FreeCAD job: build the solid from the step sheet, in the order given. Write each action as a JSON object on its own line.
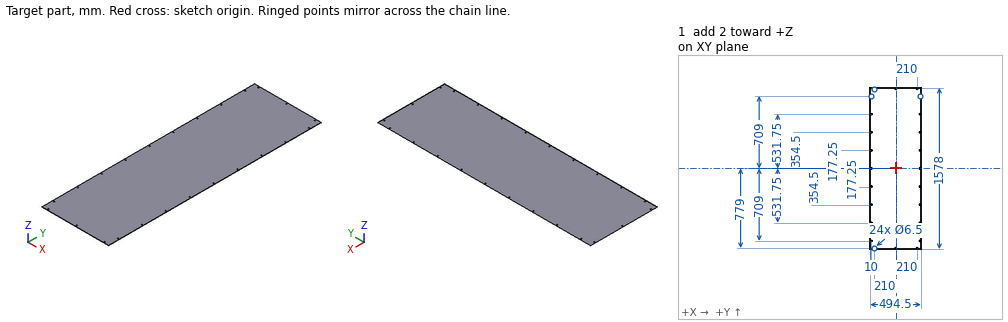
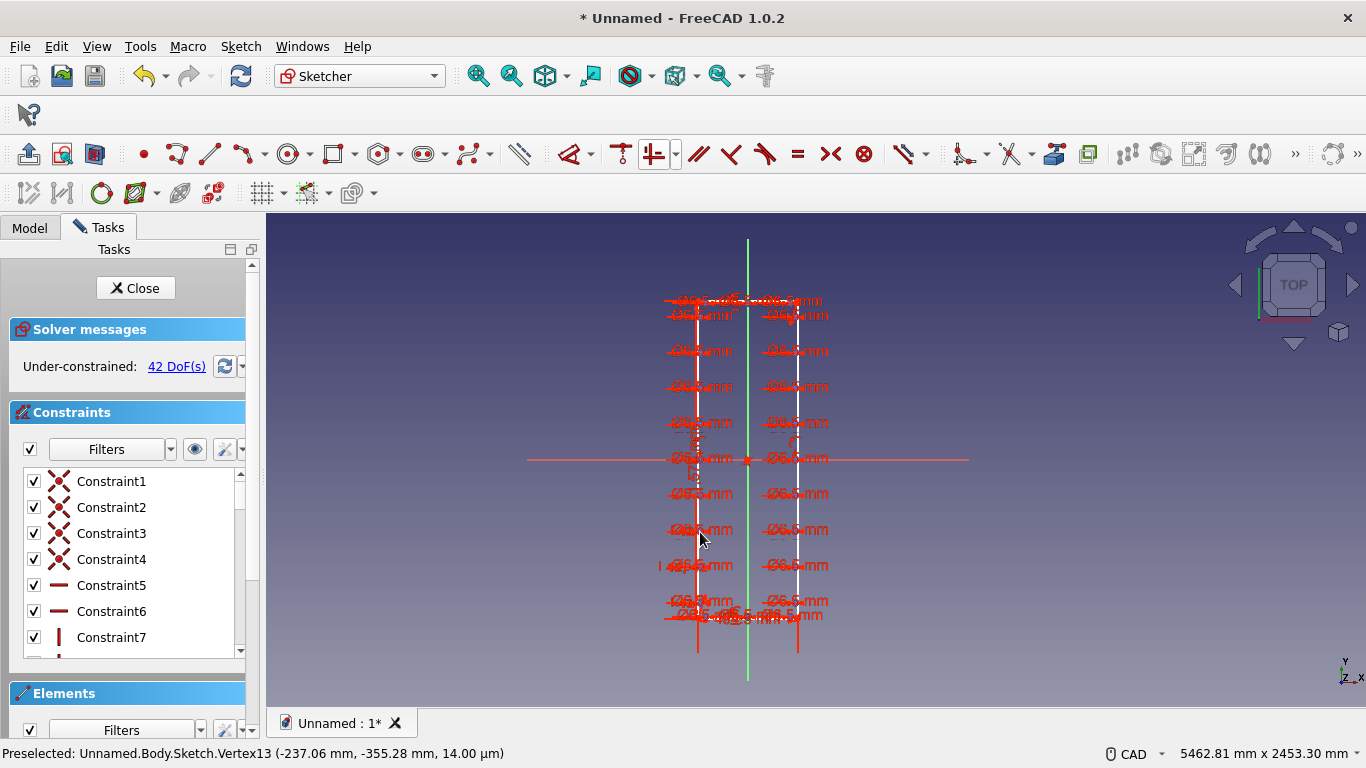
{"action": "left_click", "coordinate": [700, 532]}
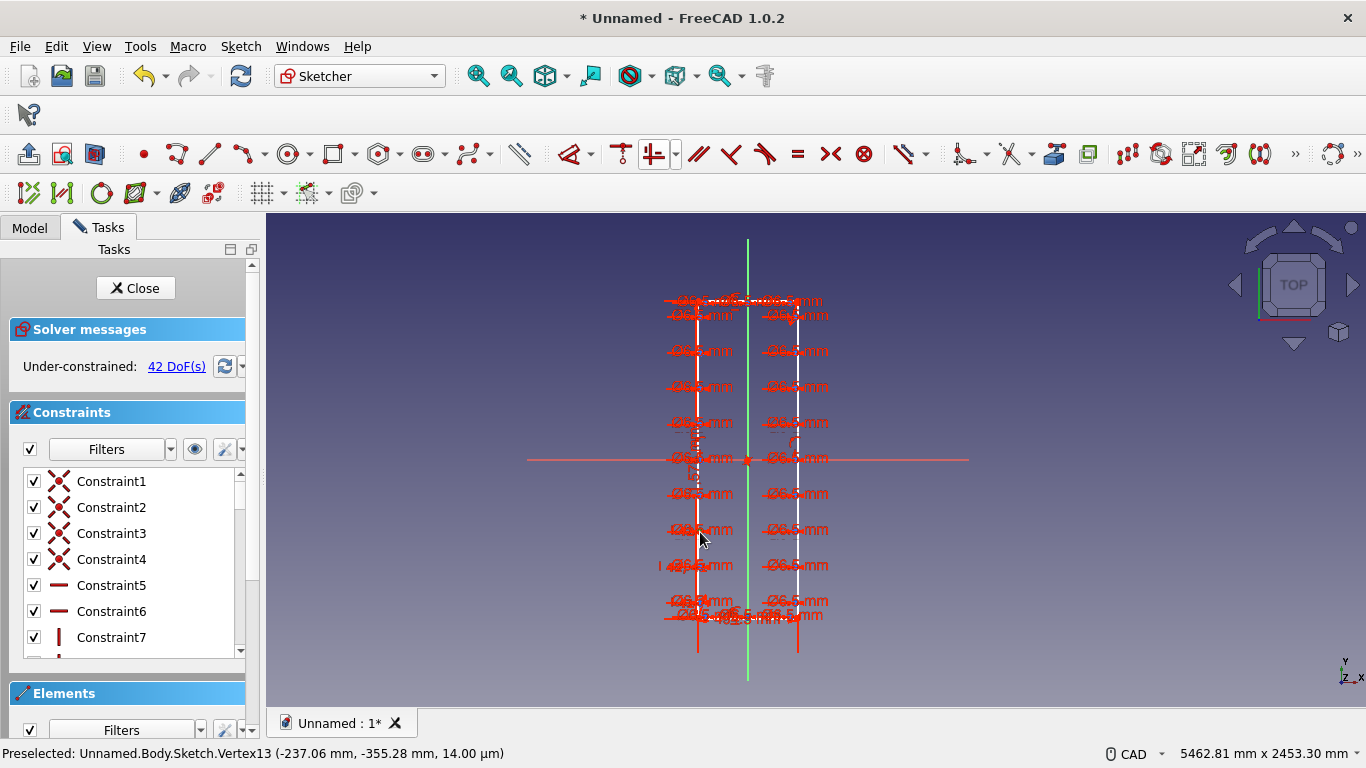
{"action": "left_click", "coordinate": [700, 496]}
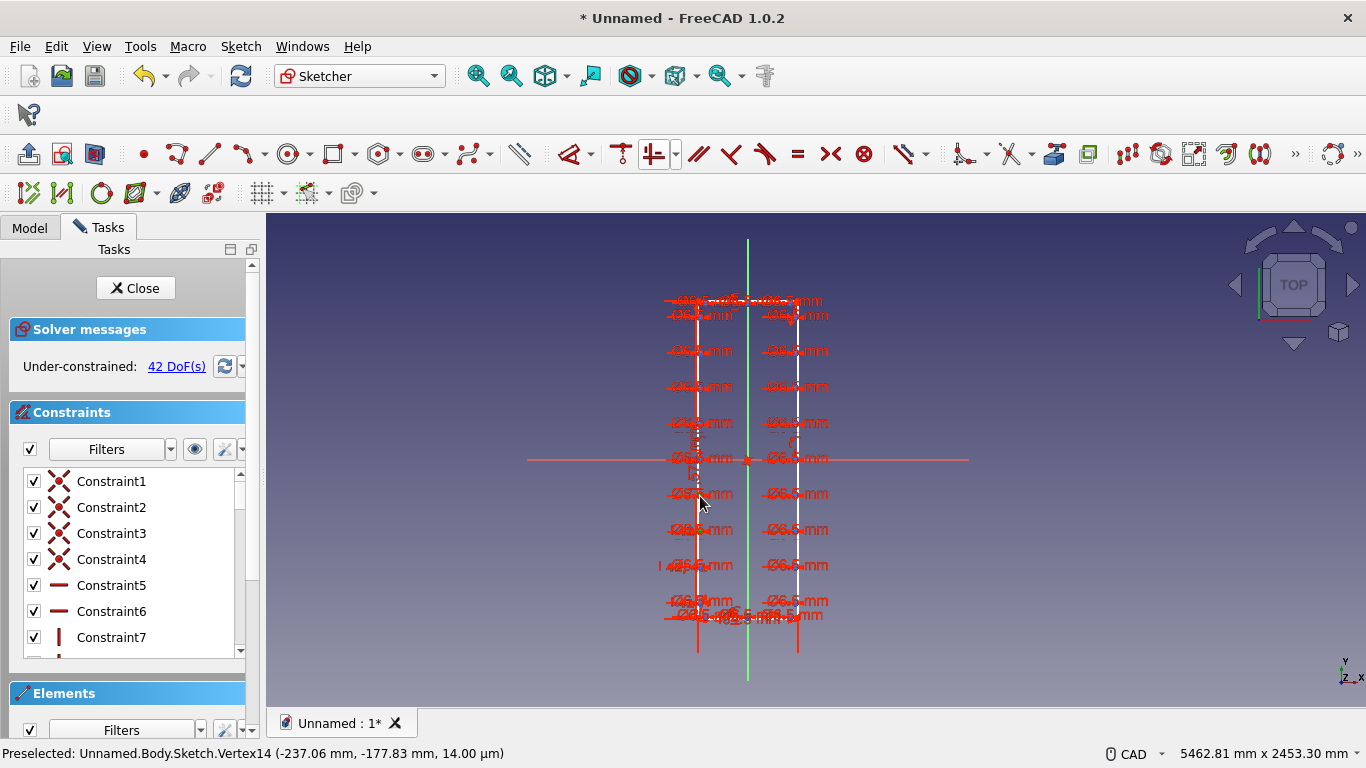
{"action": "left_click", "coordinate": [676, 154]}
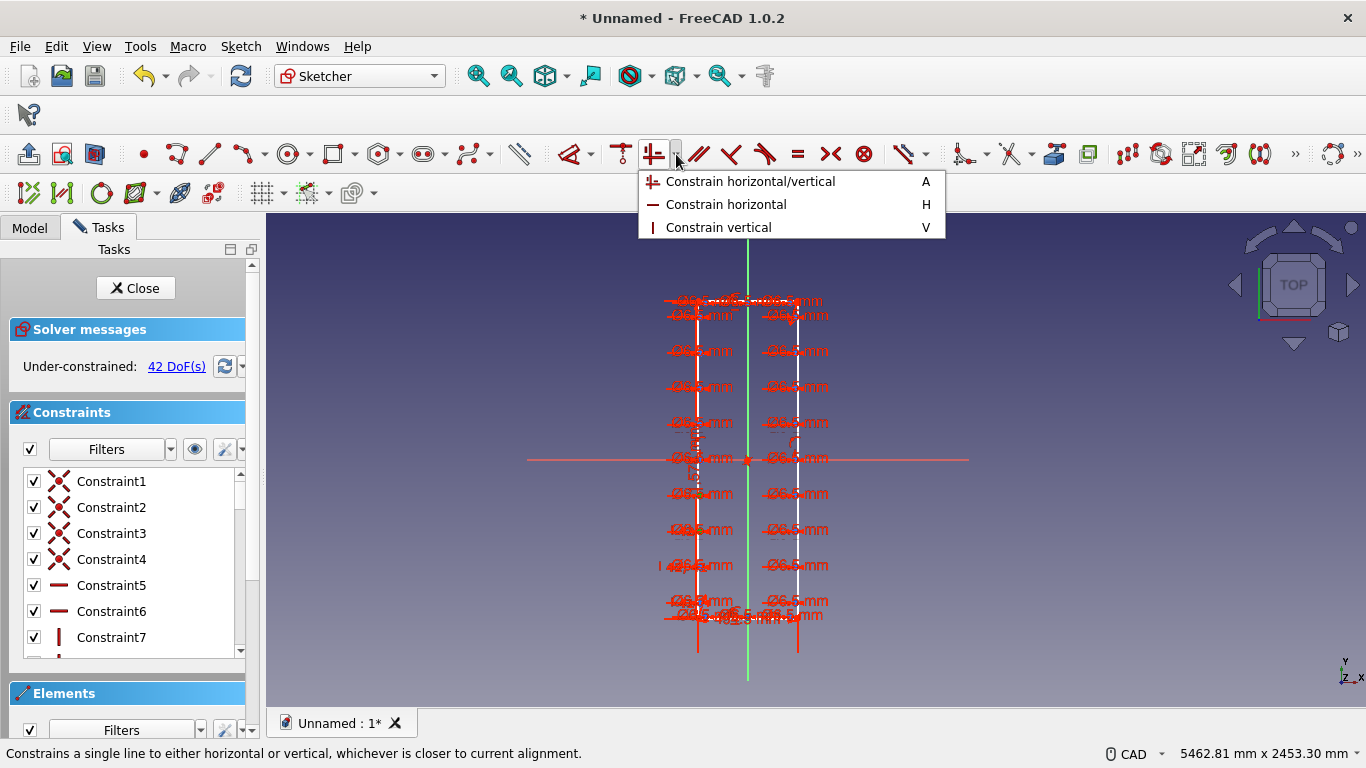
{"action": "left_click", "coordinate": [792, 228]}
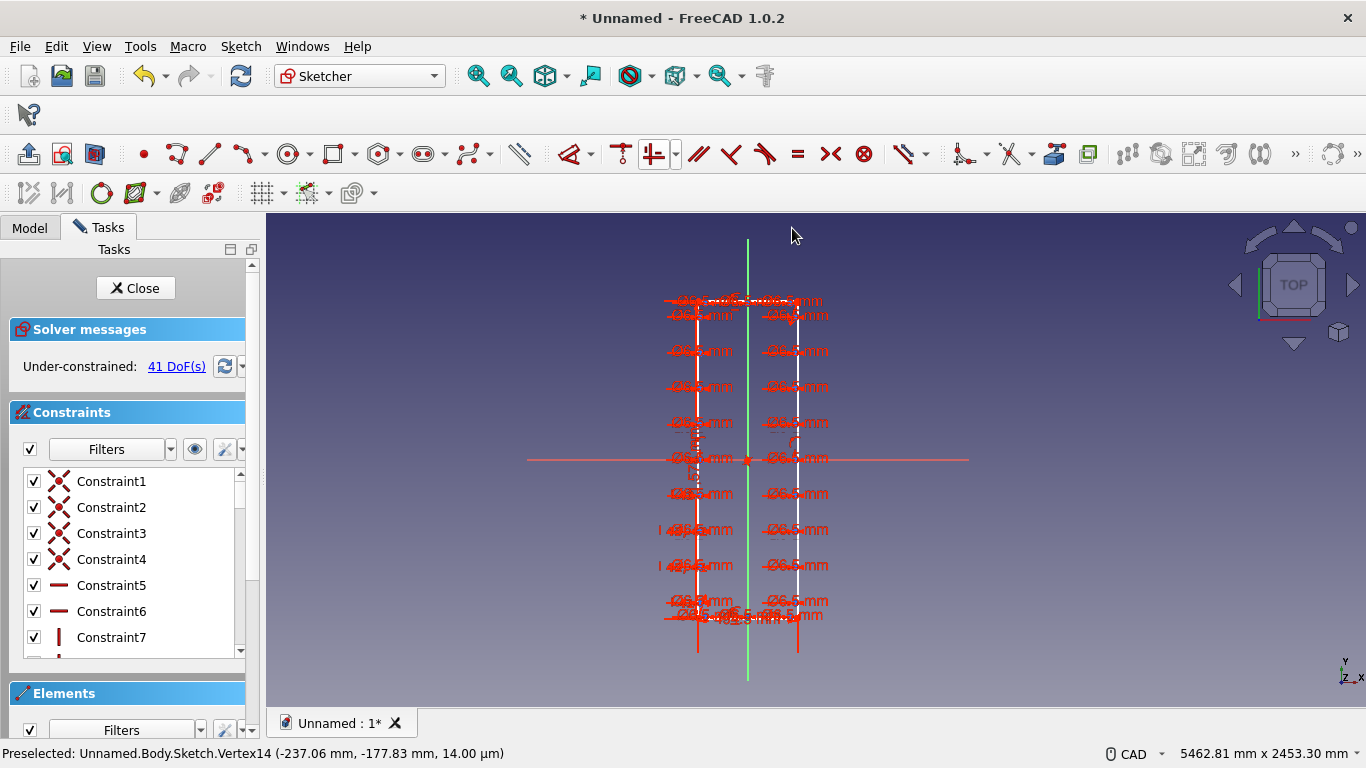
{"action": "scroll", "coordinate": [706, 617], "scroll_direction": "up", "scroll_amount": 3}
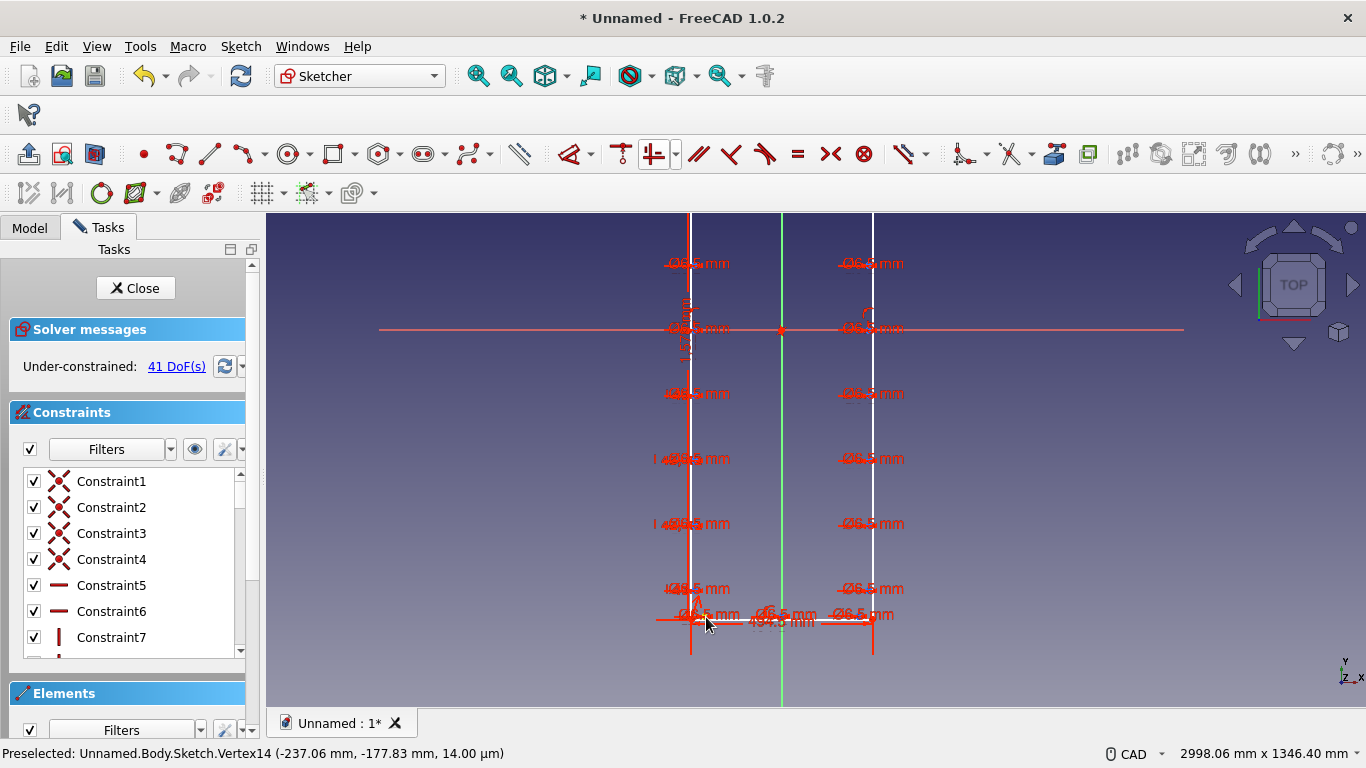
{"action": "left_click", "coordinate": [705, 617]}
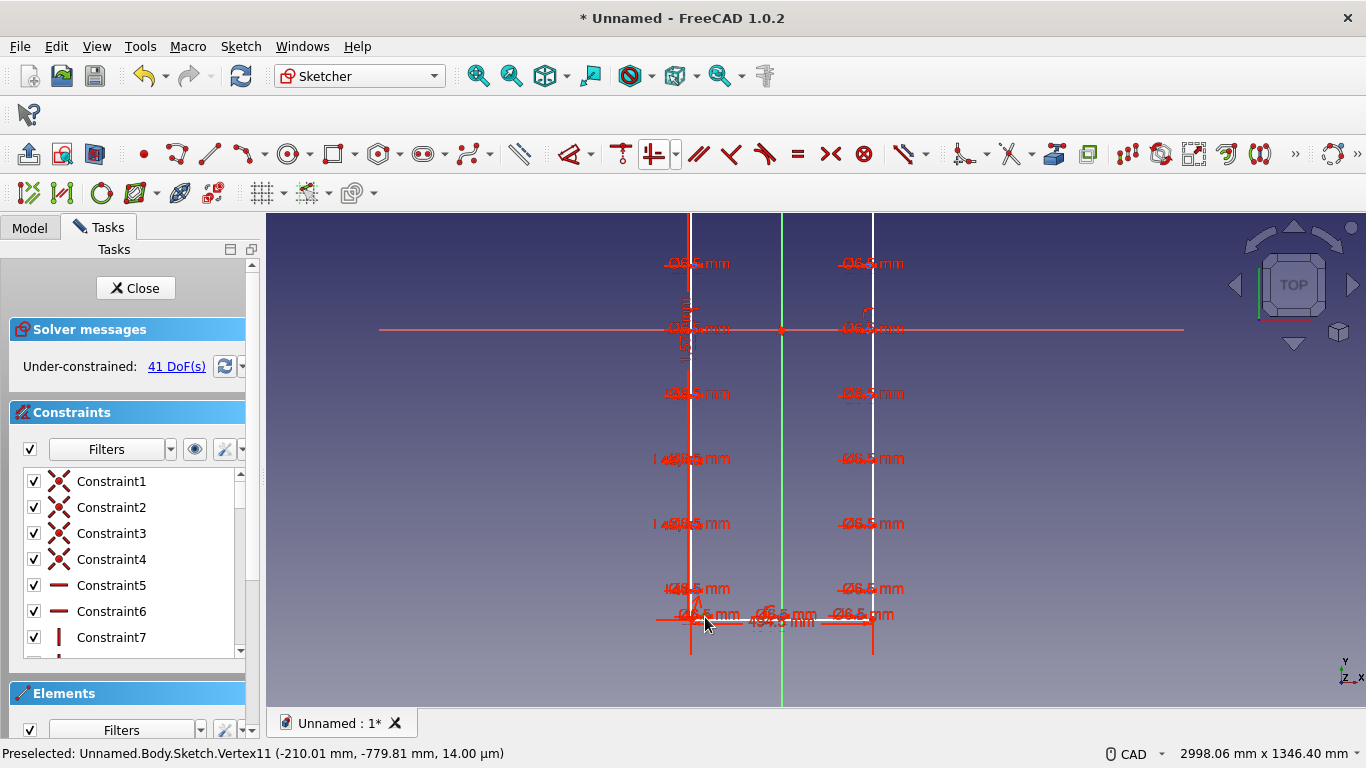
{"action": "left_click", "coordinate": [782, 617]}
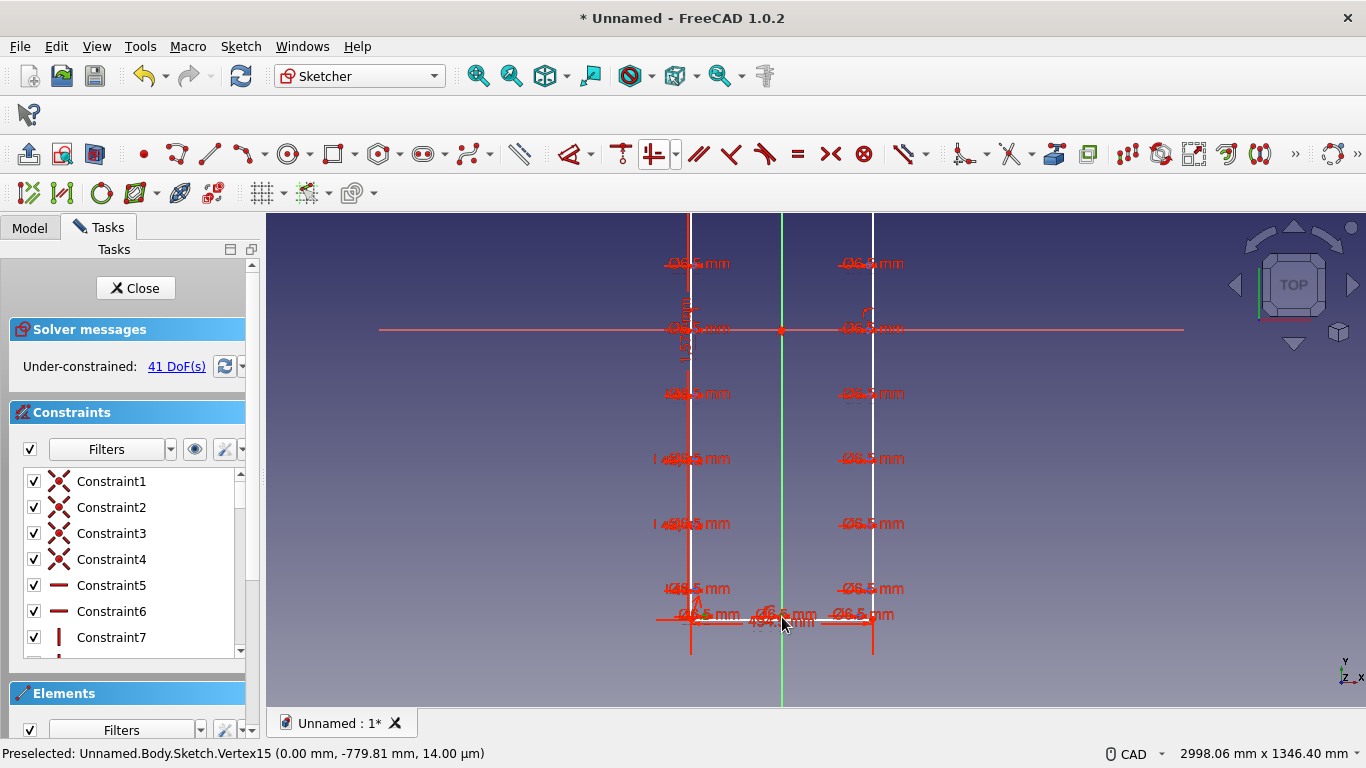
{"action": "key", "text": "h"}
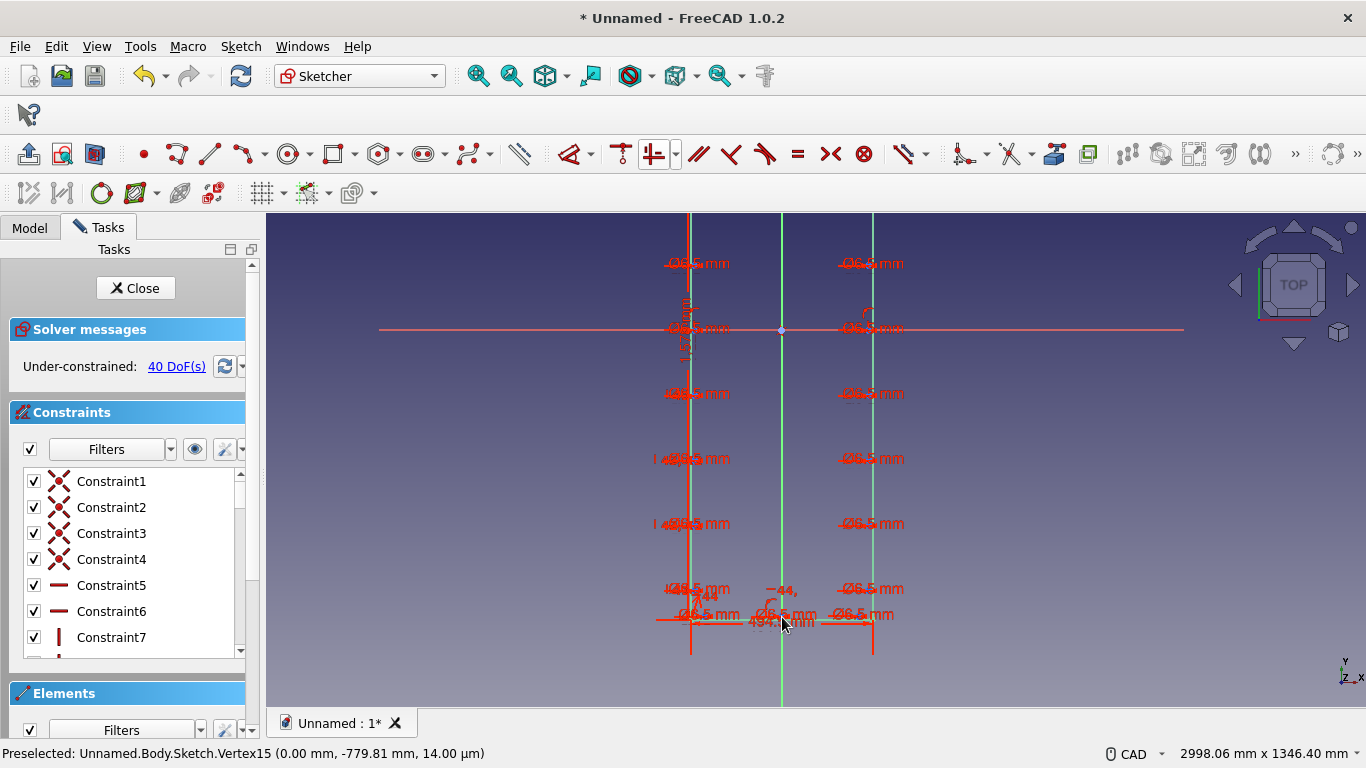
{"action": "left_click", "coordinate": [782, 617]}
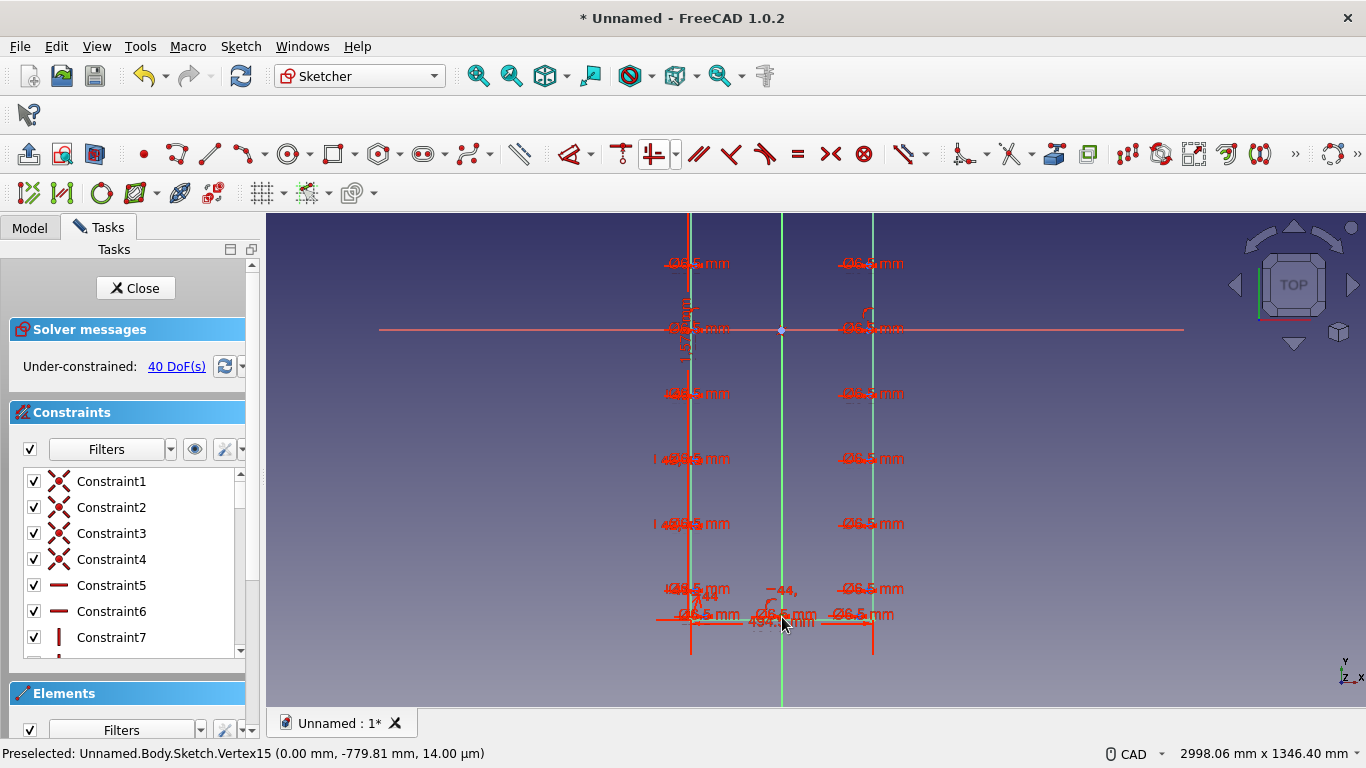
{"action": "left_click", "coordinate": [859, 616]}